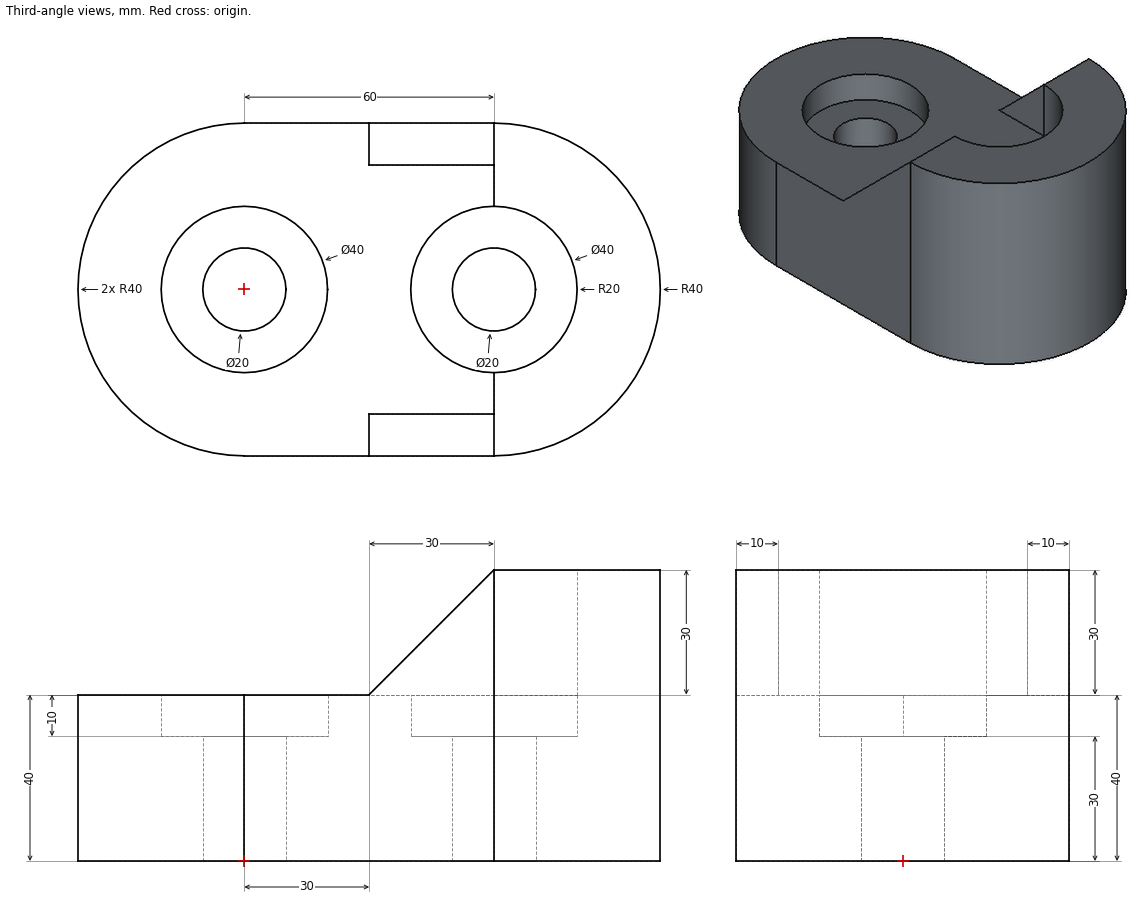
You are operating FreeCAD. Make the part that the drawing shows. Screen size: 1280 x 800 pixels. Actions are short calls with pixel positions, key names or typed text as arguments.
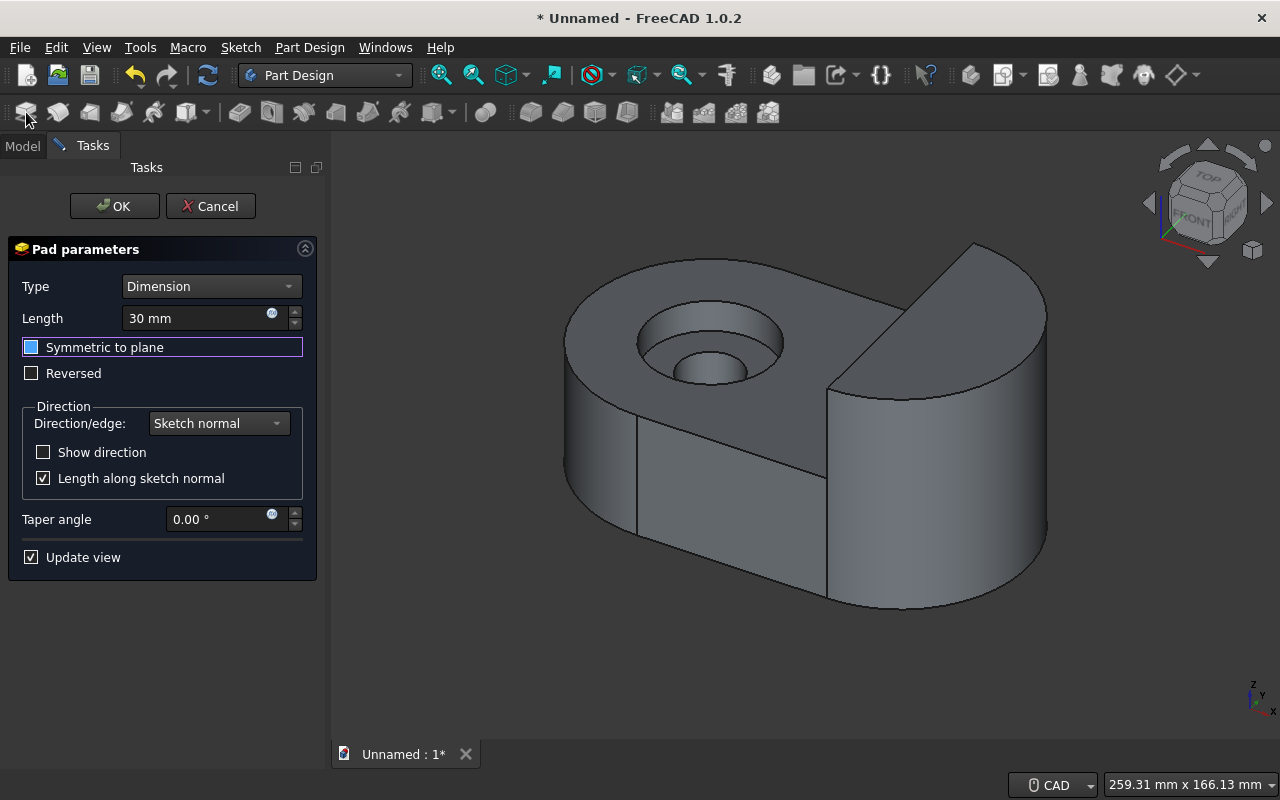
click(115, 206)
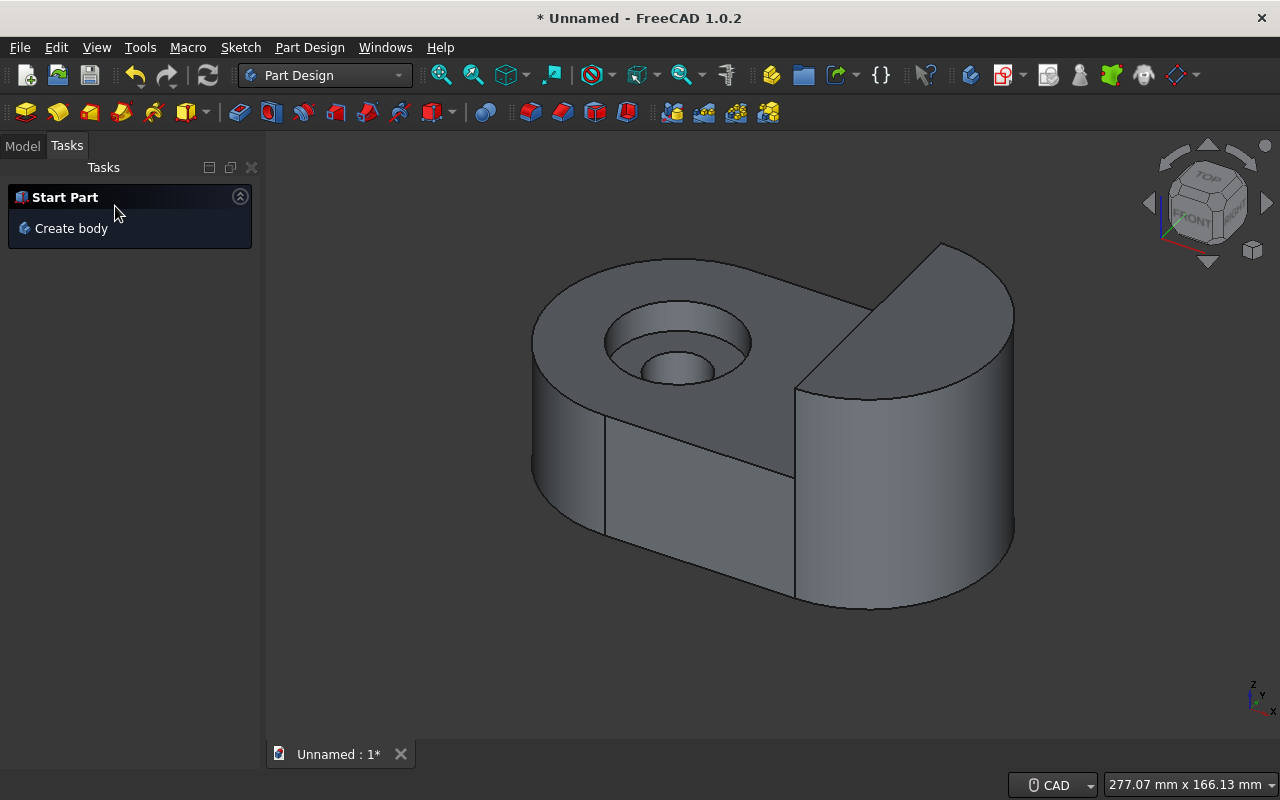
click(931, 336)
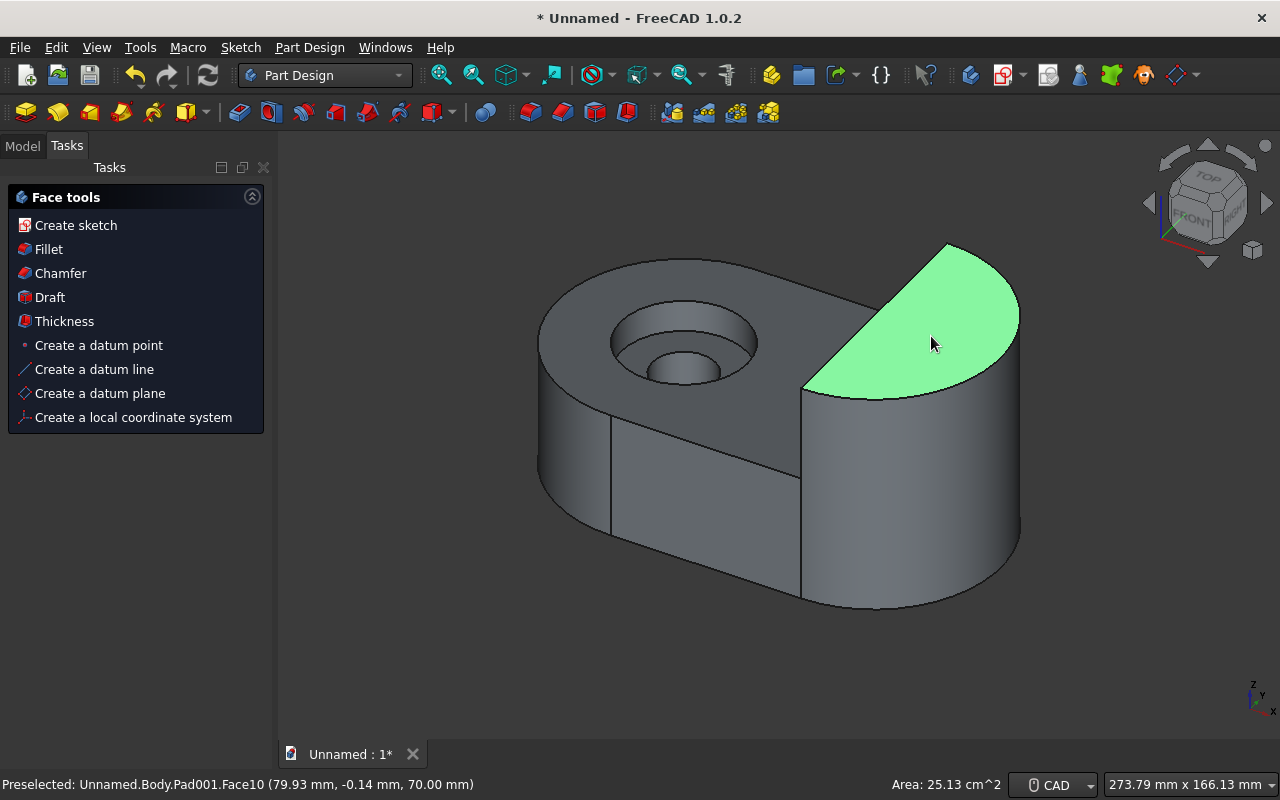
click(1004, 76)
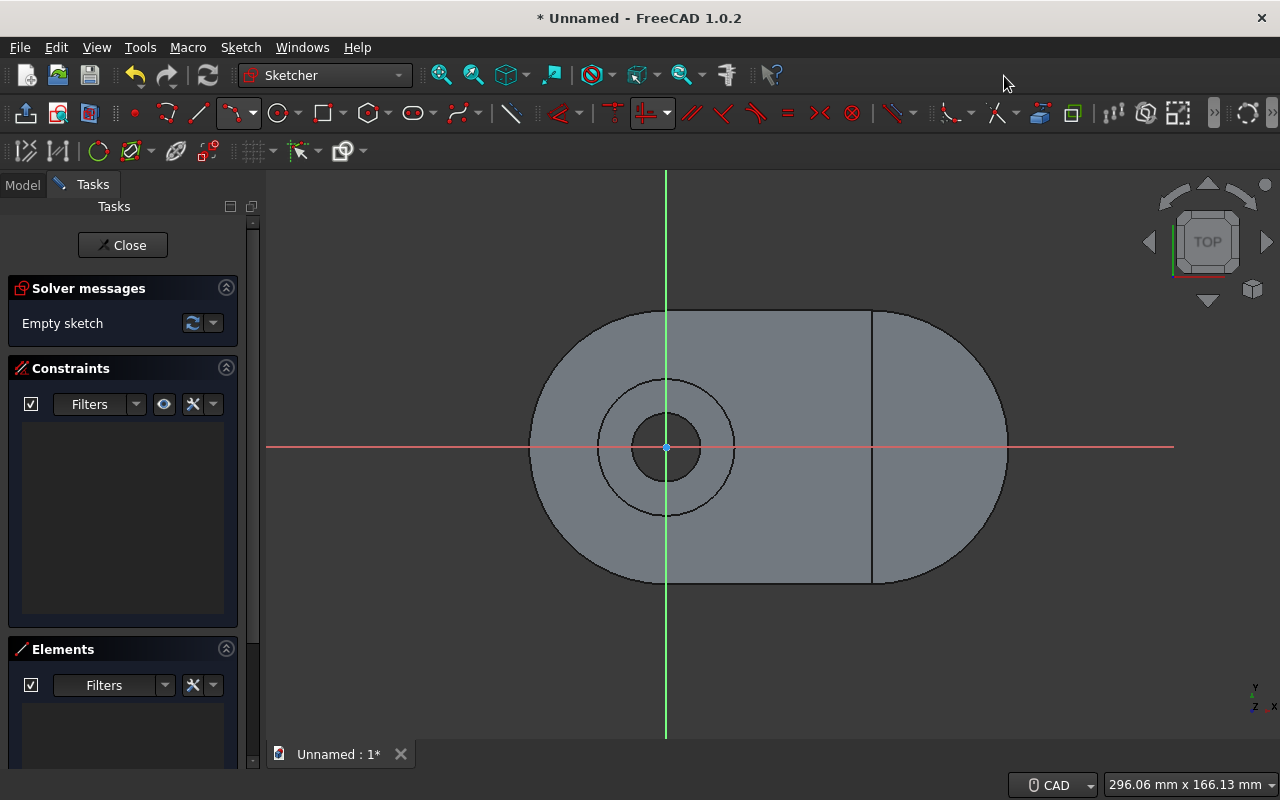
scroll(884, 442, up, 4)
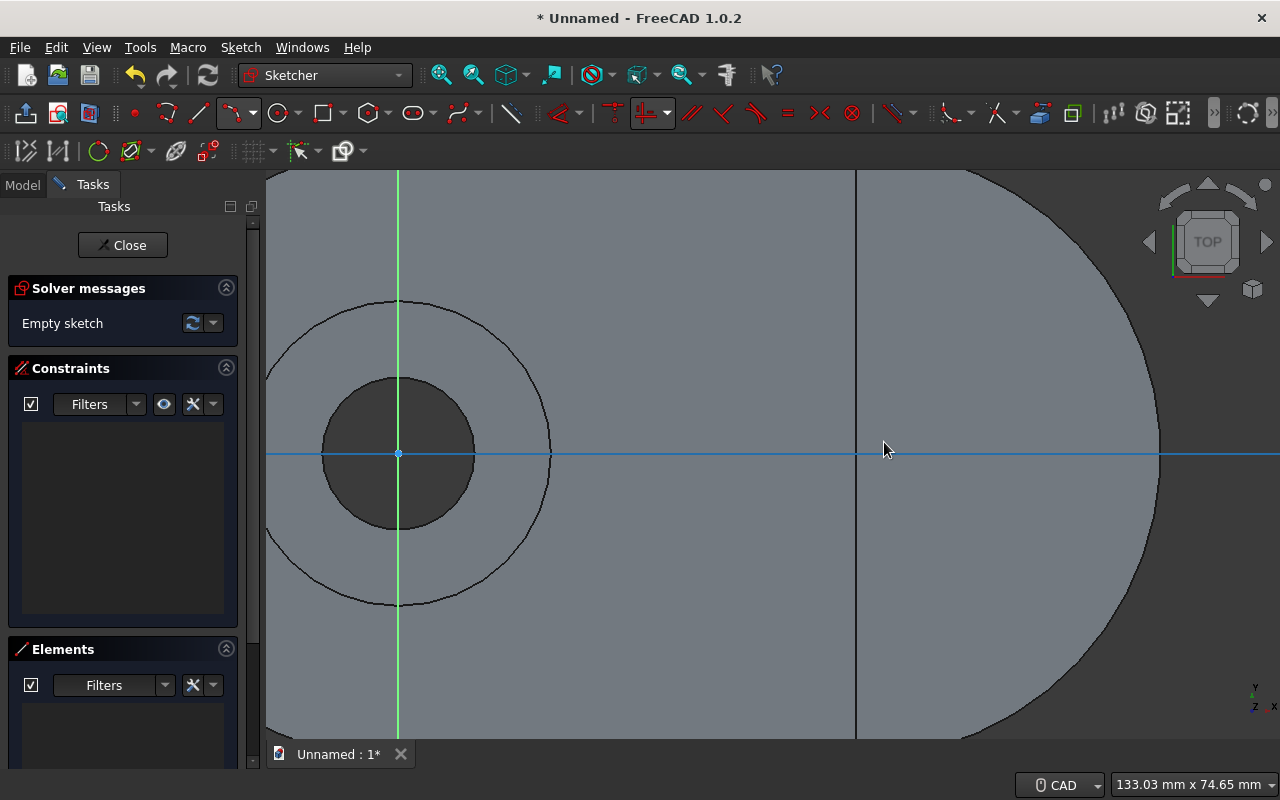
click(200, 114)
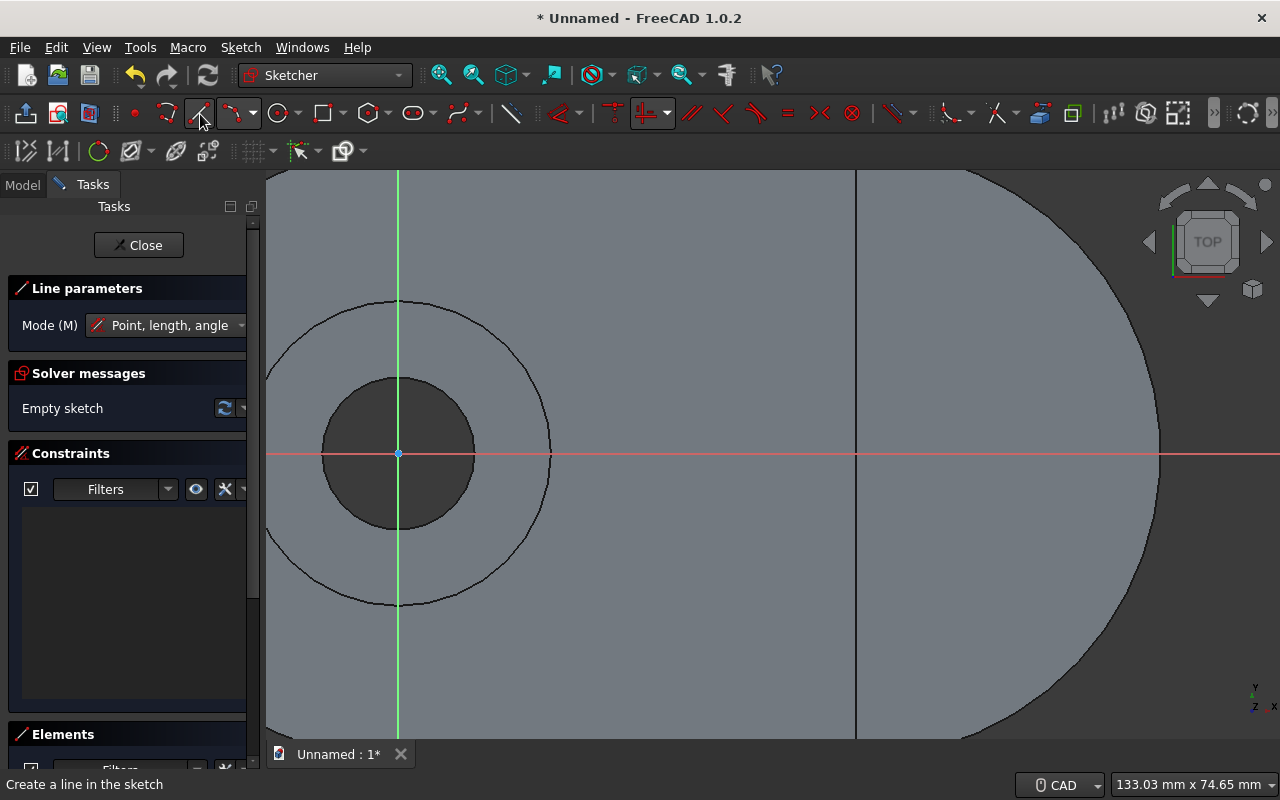
click(856, 301)
click(856, 606)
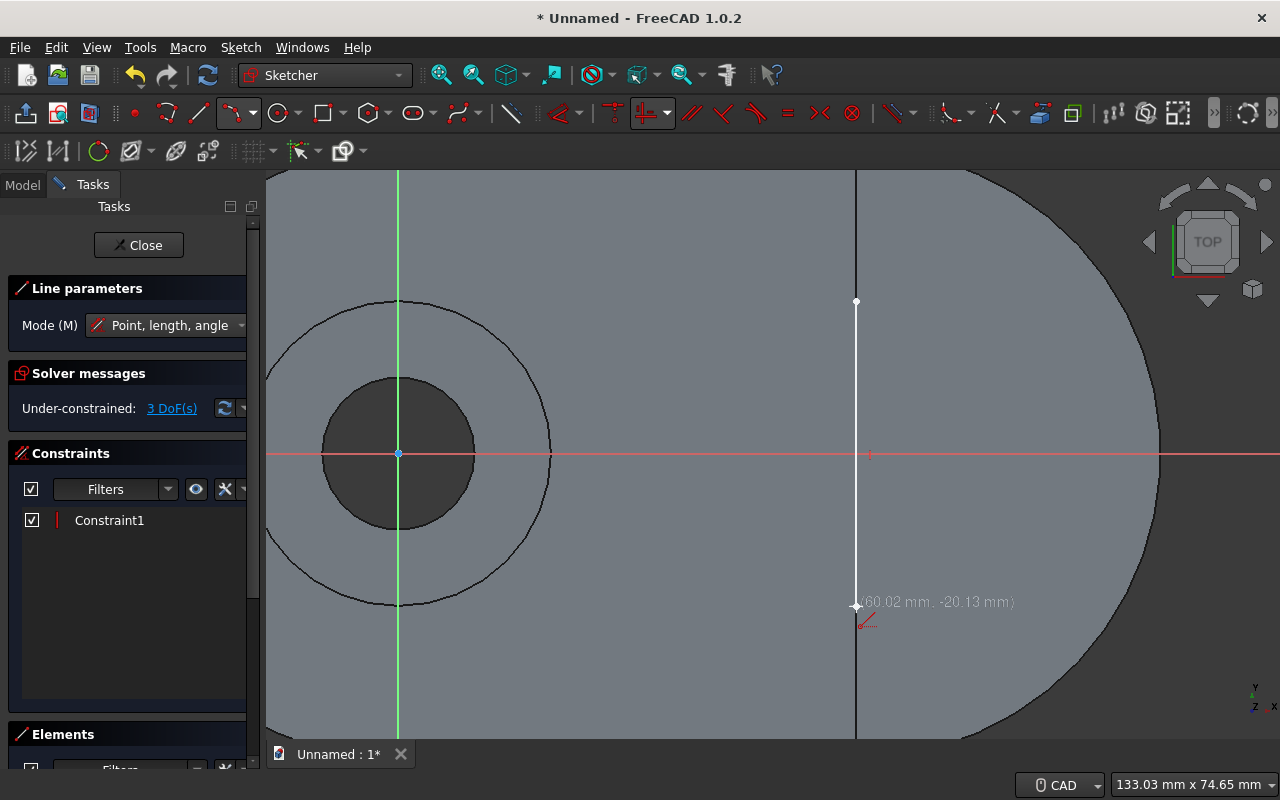
click(232, 114)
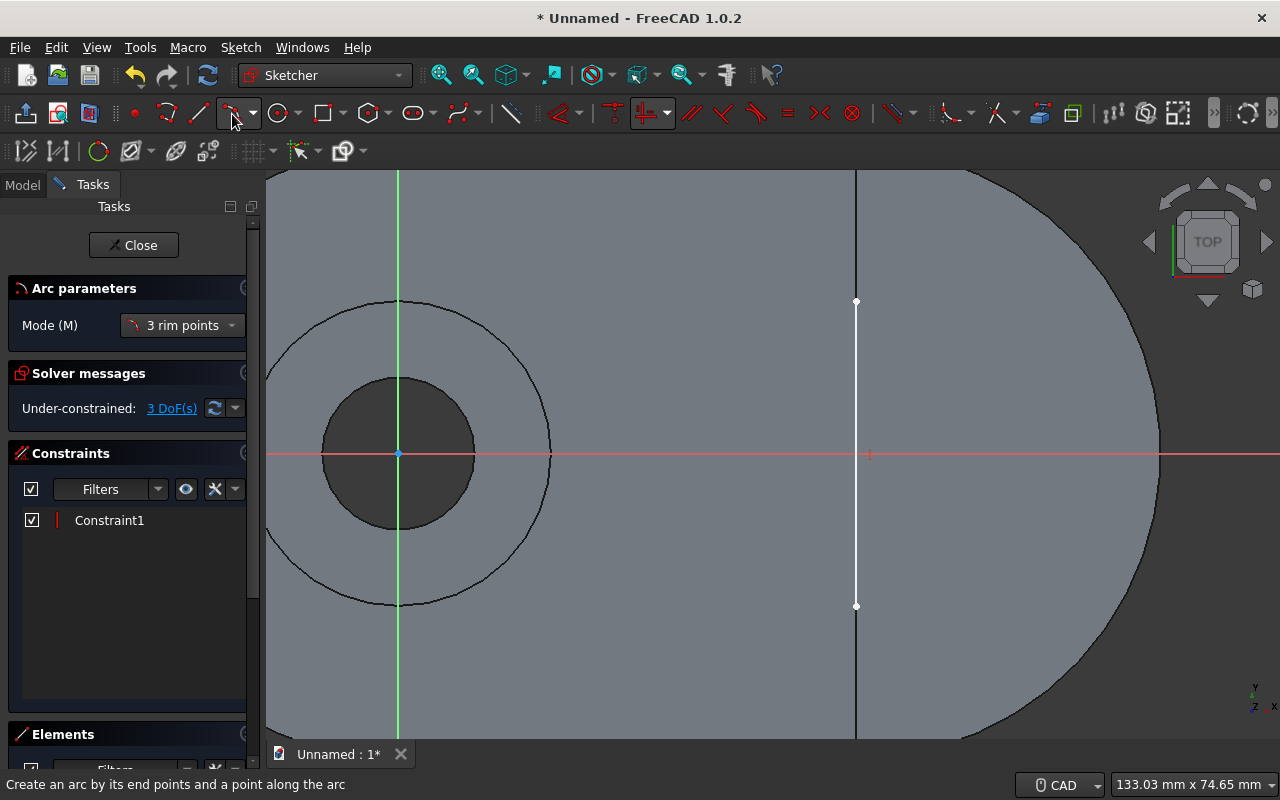
click(856, 607)
click(856, 302)
click(1001, 501)
key(Escape)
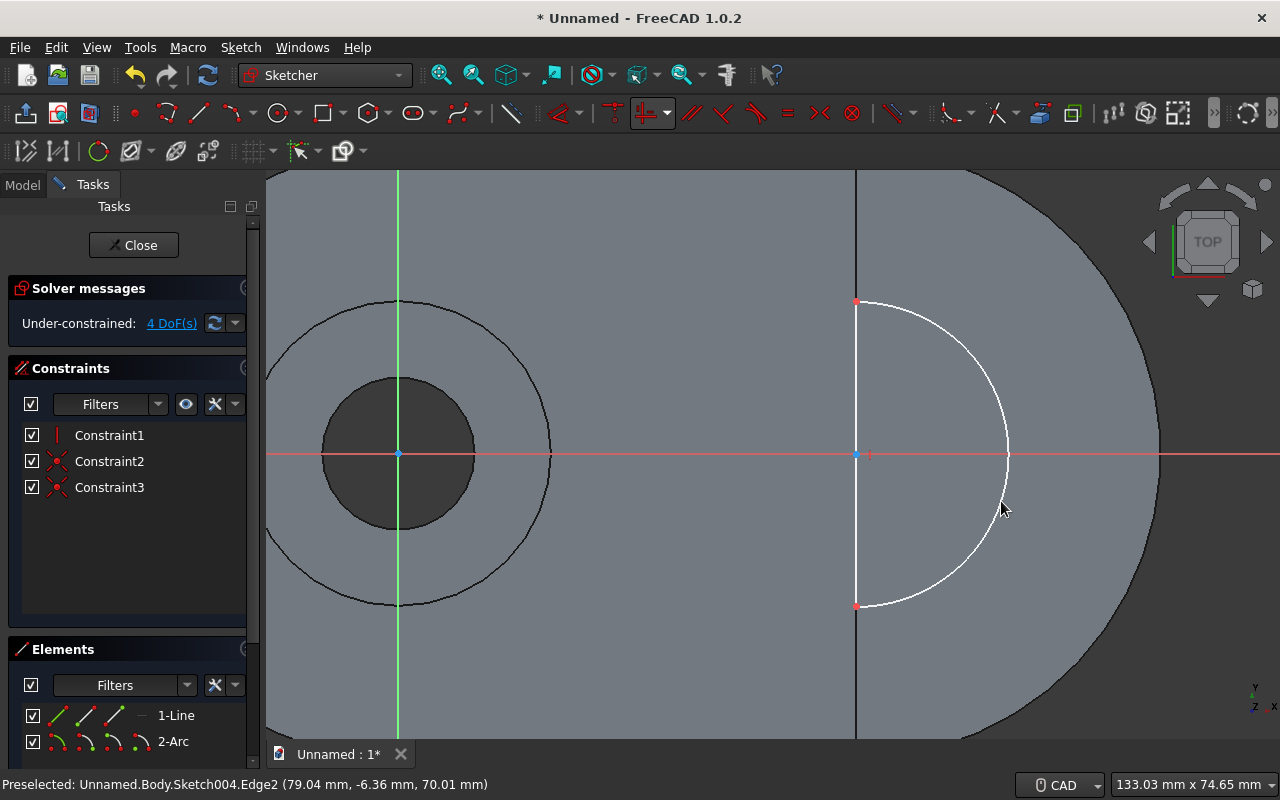
click(856, 454)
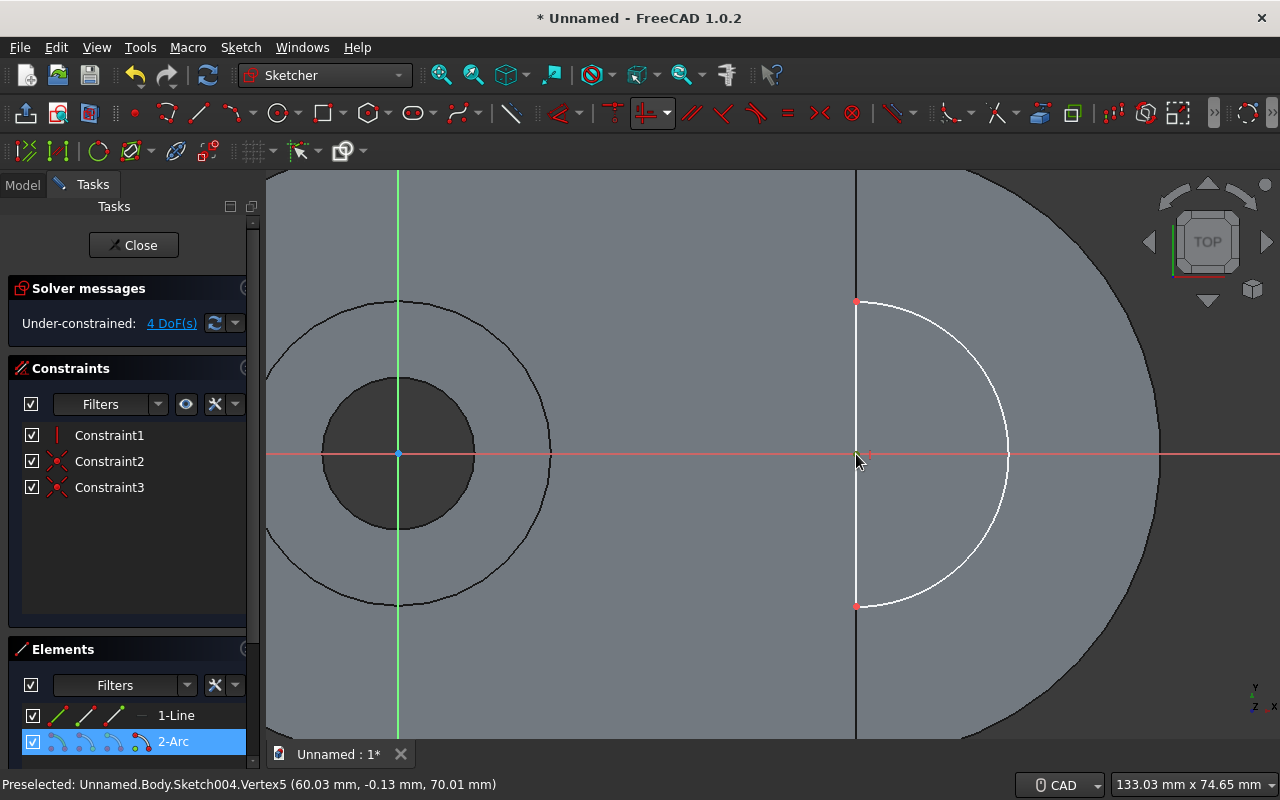
click(353, 454)